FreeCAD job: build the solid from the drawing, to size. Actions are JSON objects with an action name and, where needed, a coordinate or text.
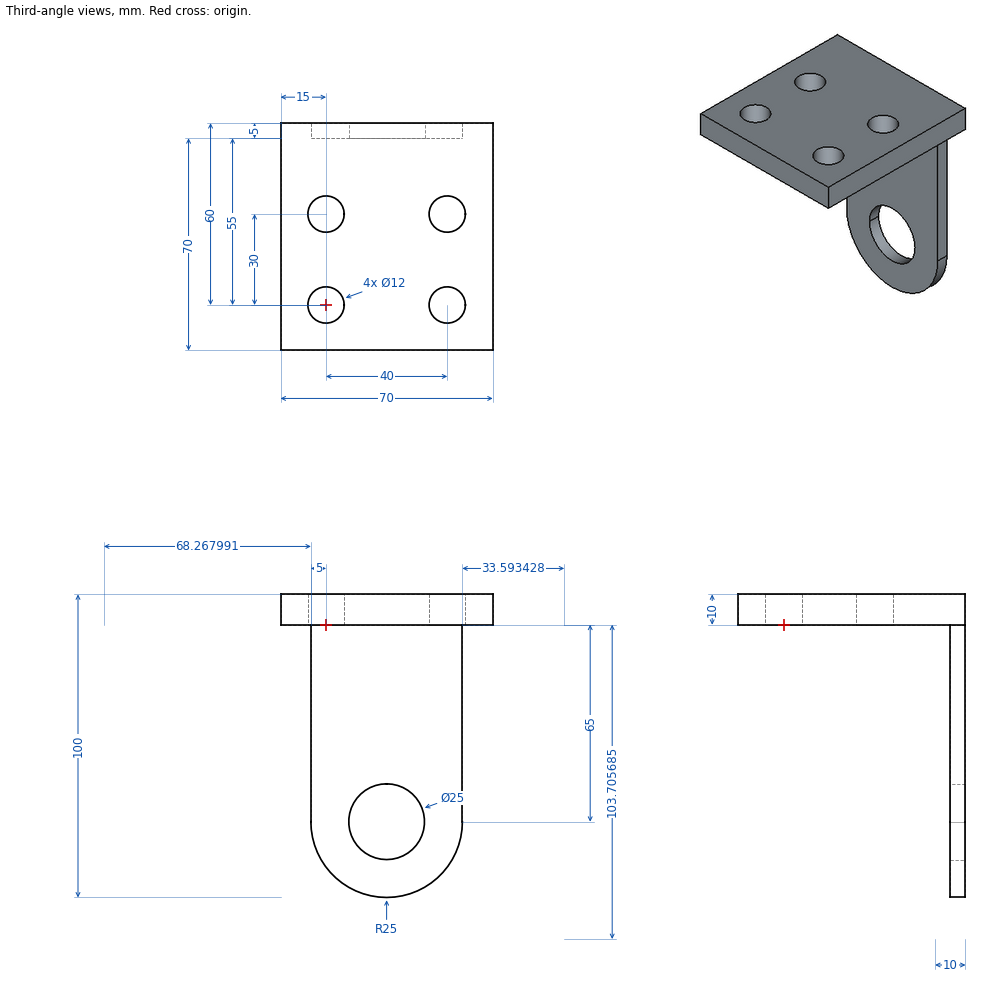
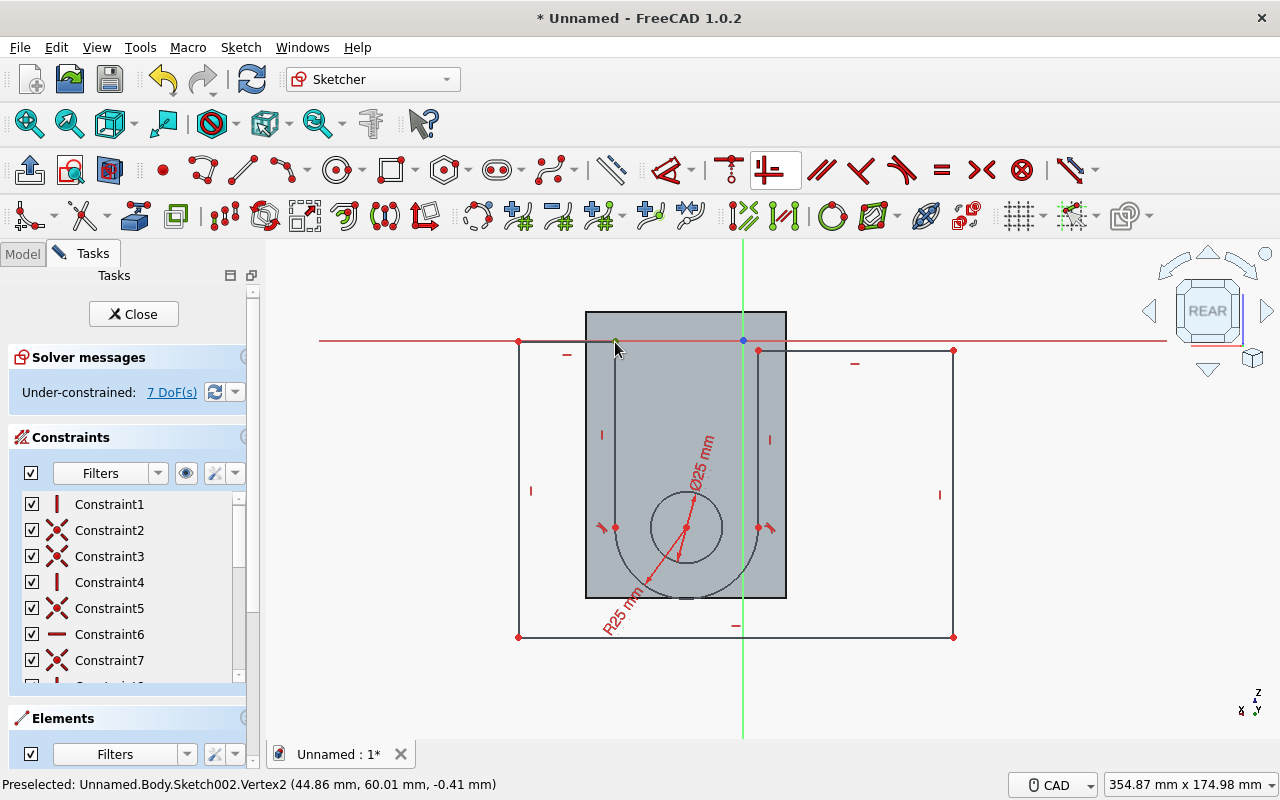
{"action": "left_click", "coordinate": [353, 341]}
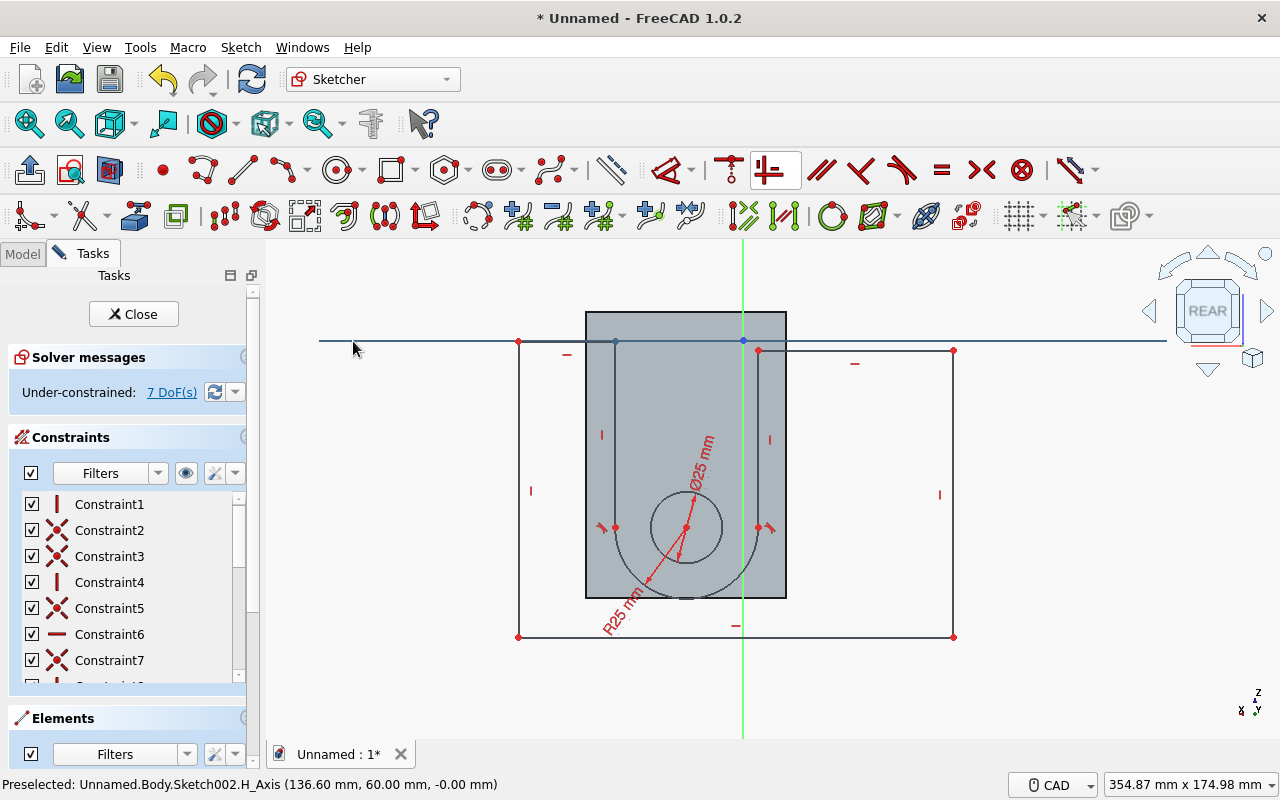
{"action": "left_click", "coordinate": [730, 170]}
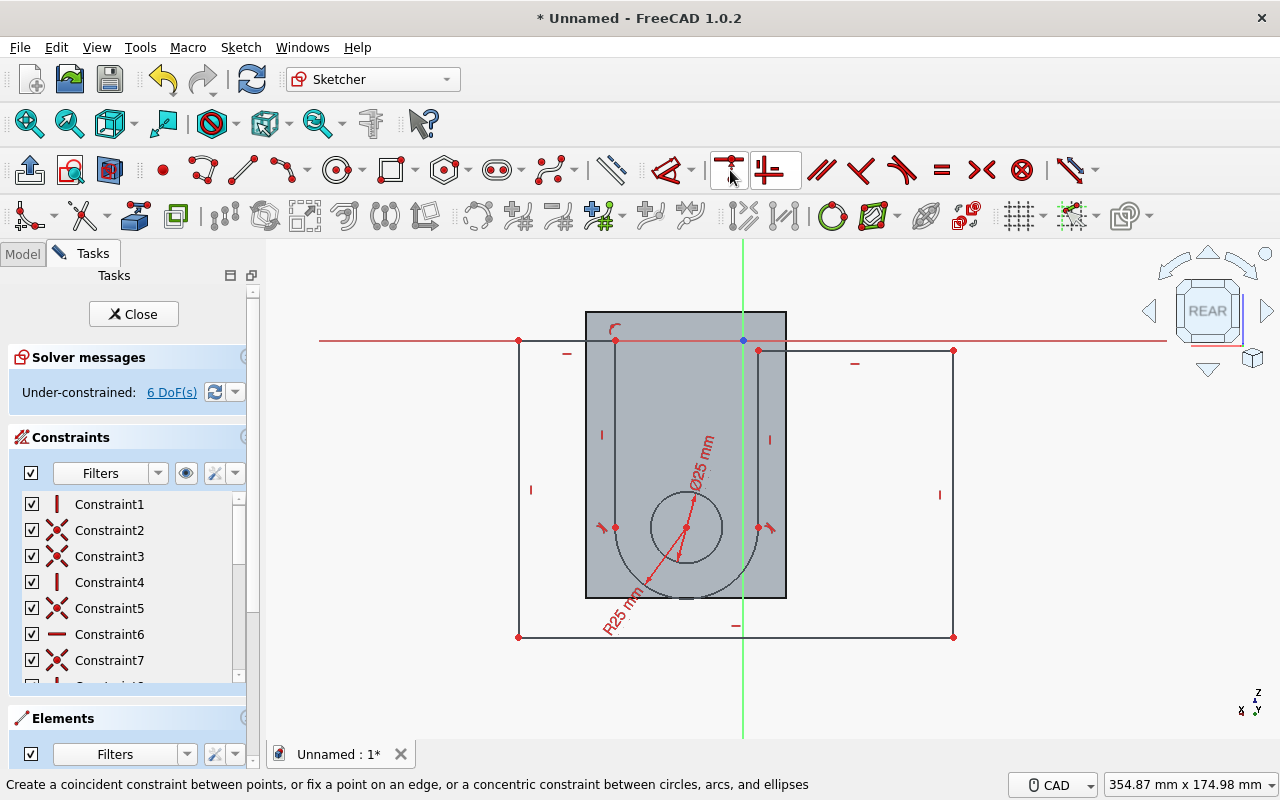
{"action": "left_click", "coordinate": [953, 351]}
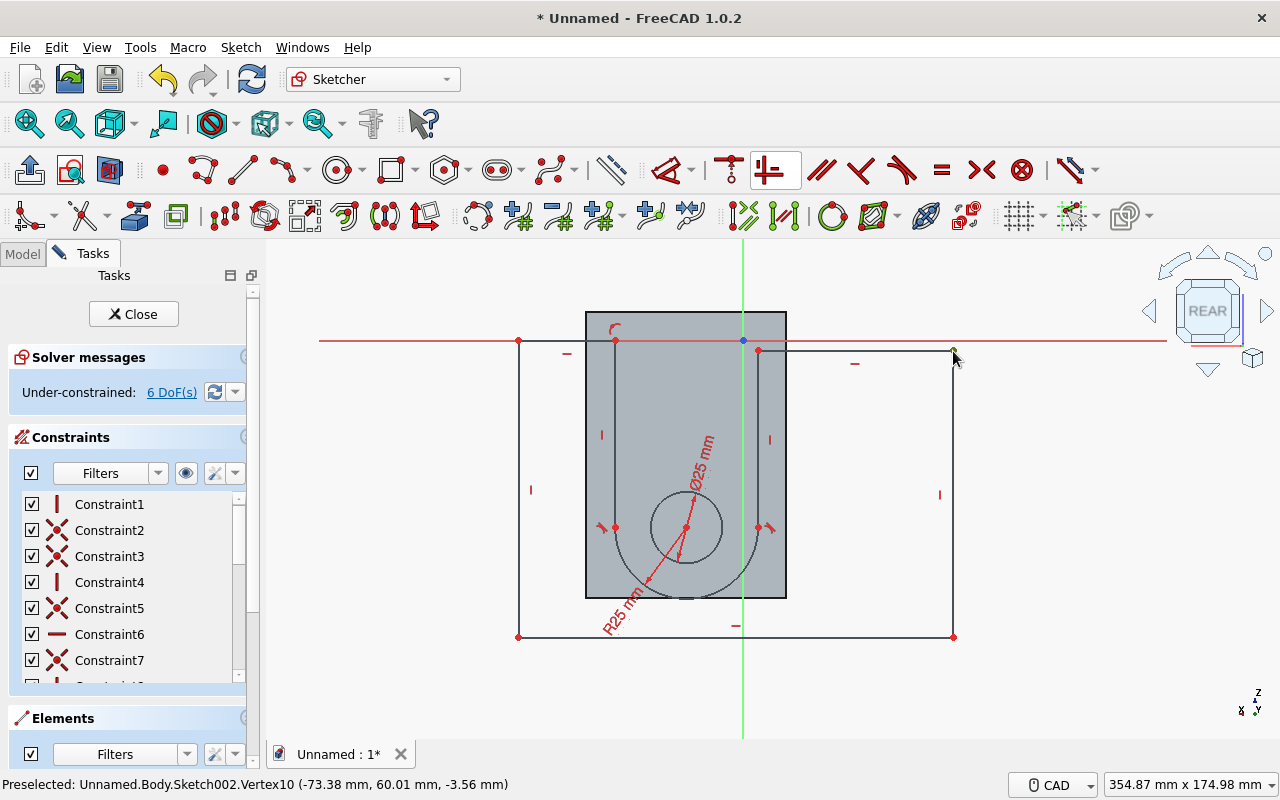
{"action": "left_click", "coordinate": [353, 341]}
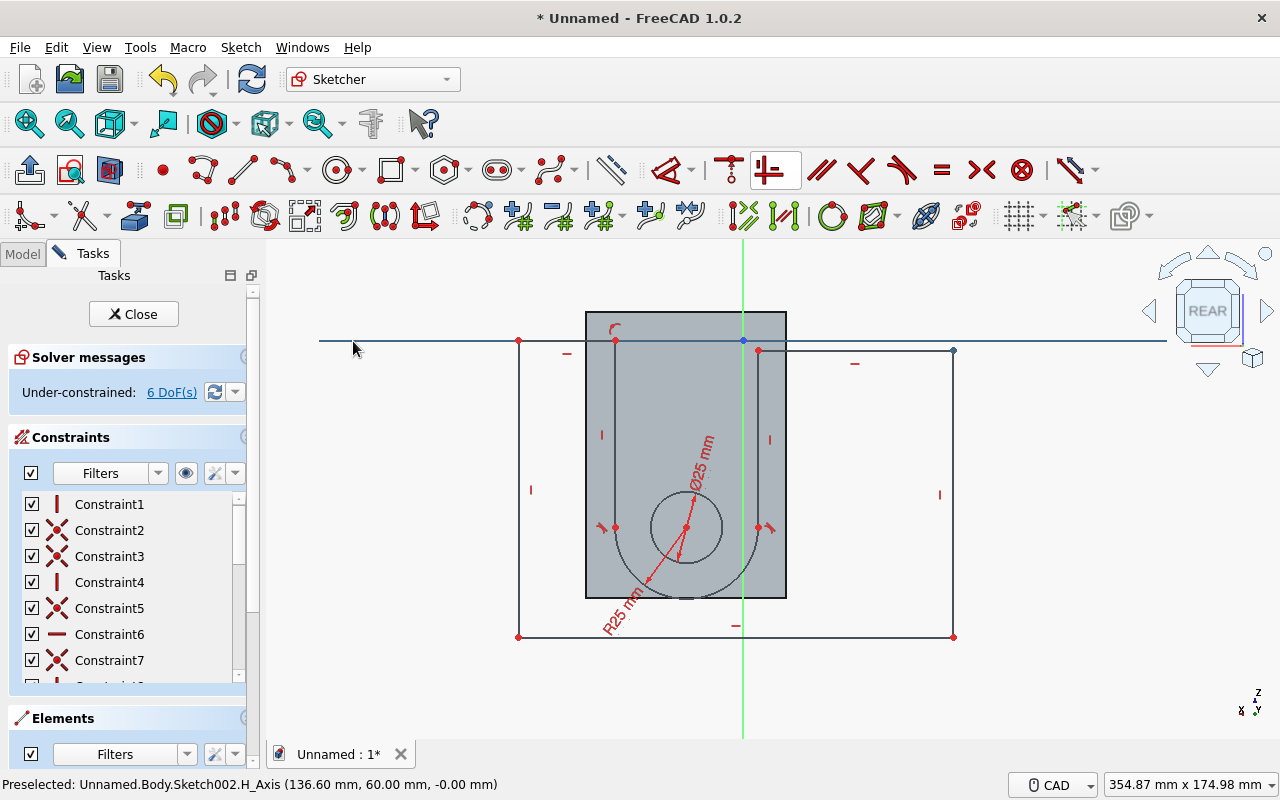
{"action": "left_click", "coordinate": [730, 170]}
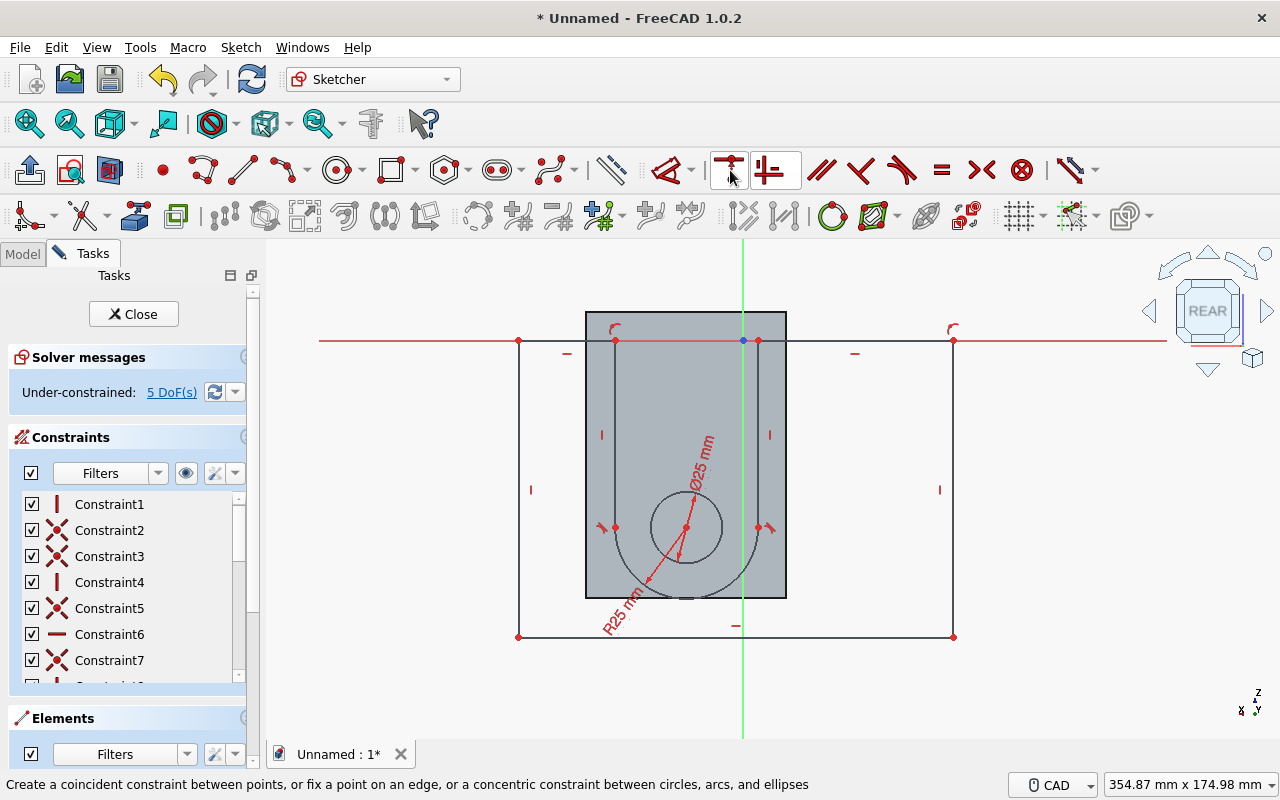
{"action": "left_click", "coordinate": [666, 170]}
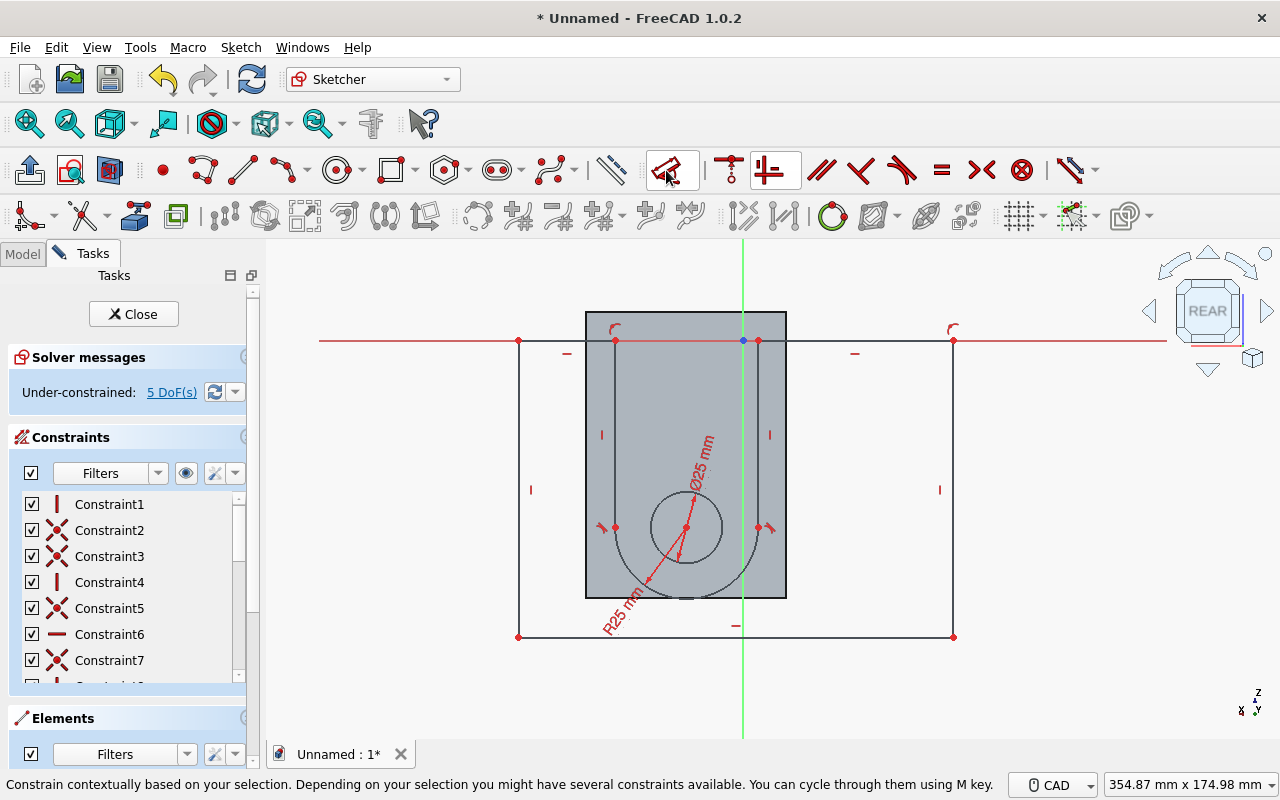
{"action": "left_click", "coordinate": [615, 471]}
{"action": "left_click", "coordinate": [581, 434]}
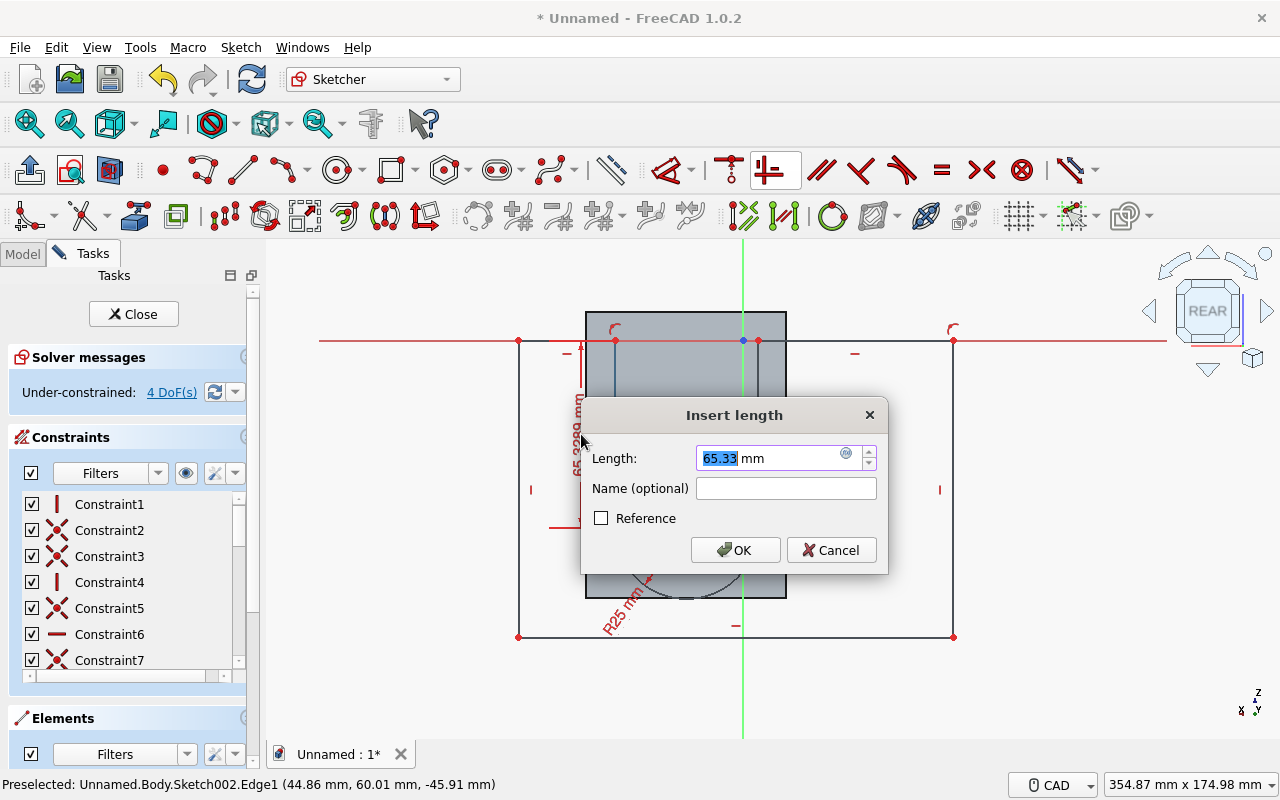
{"action": "type", "text": "65"}
{"action": "key", "text": "Return"}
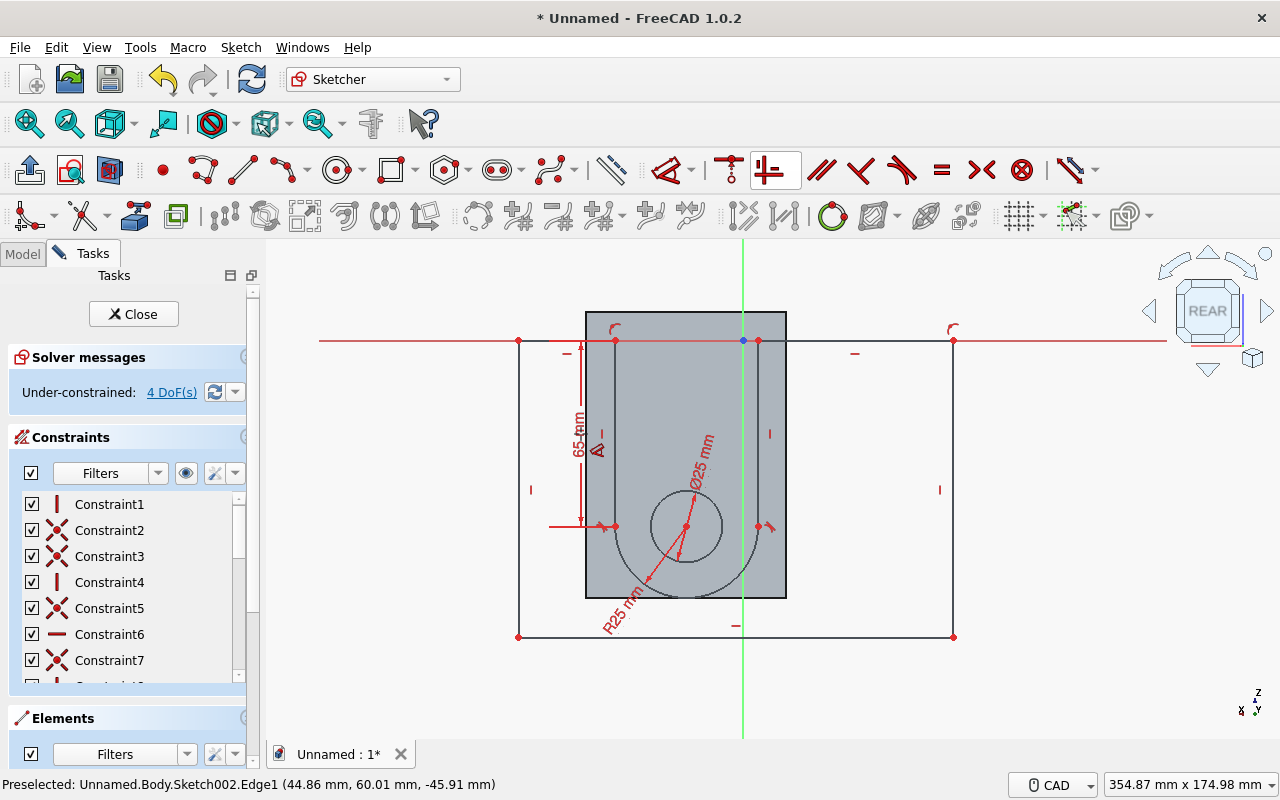
{"action": "scroll", "coordinate": [758, 341], "scroll_direction": "up", "scroll_amount": 6}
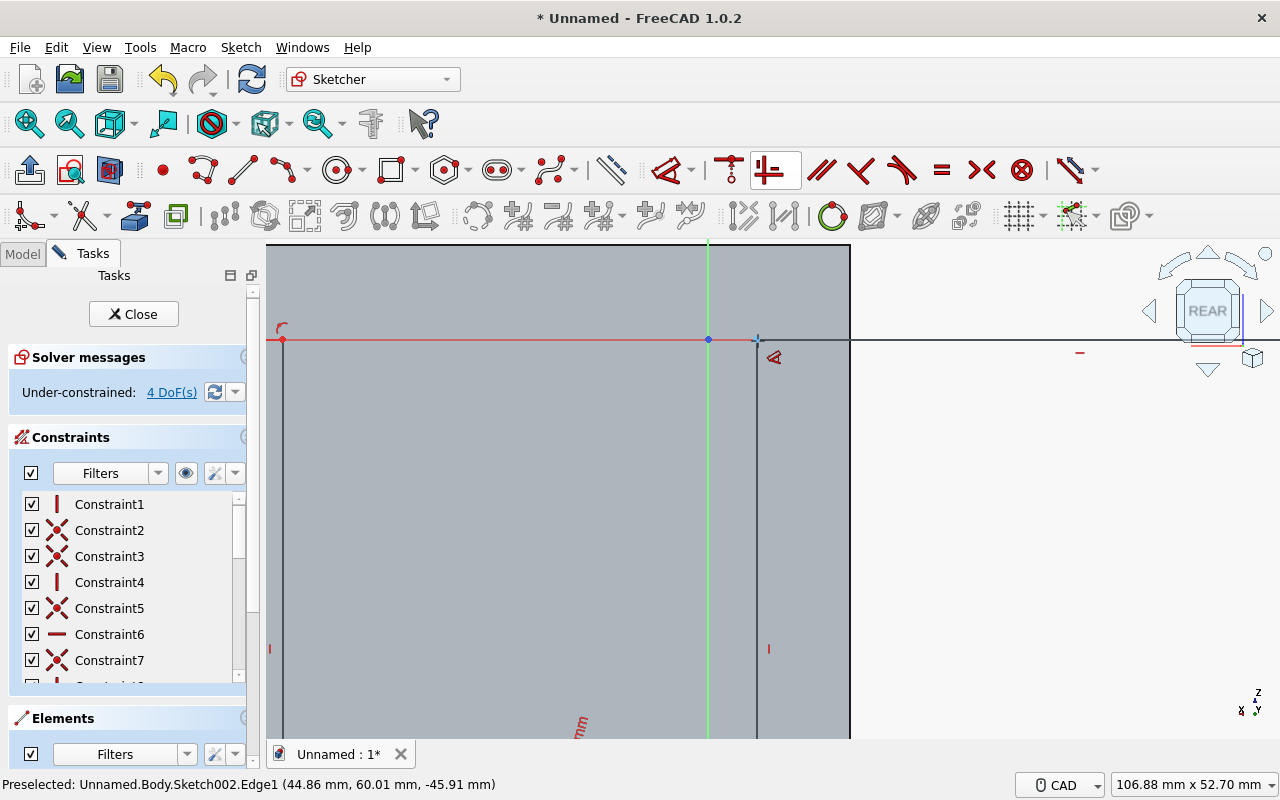
{"action": "left_click", "coordinate": [757, 340]}
{"action": "left_click", "coordinate": [733, 306]}